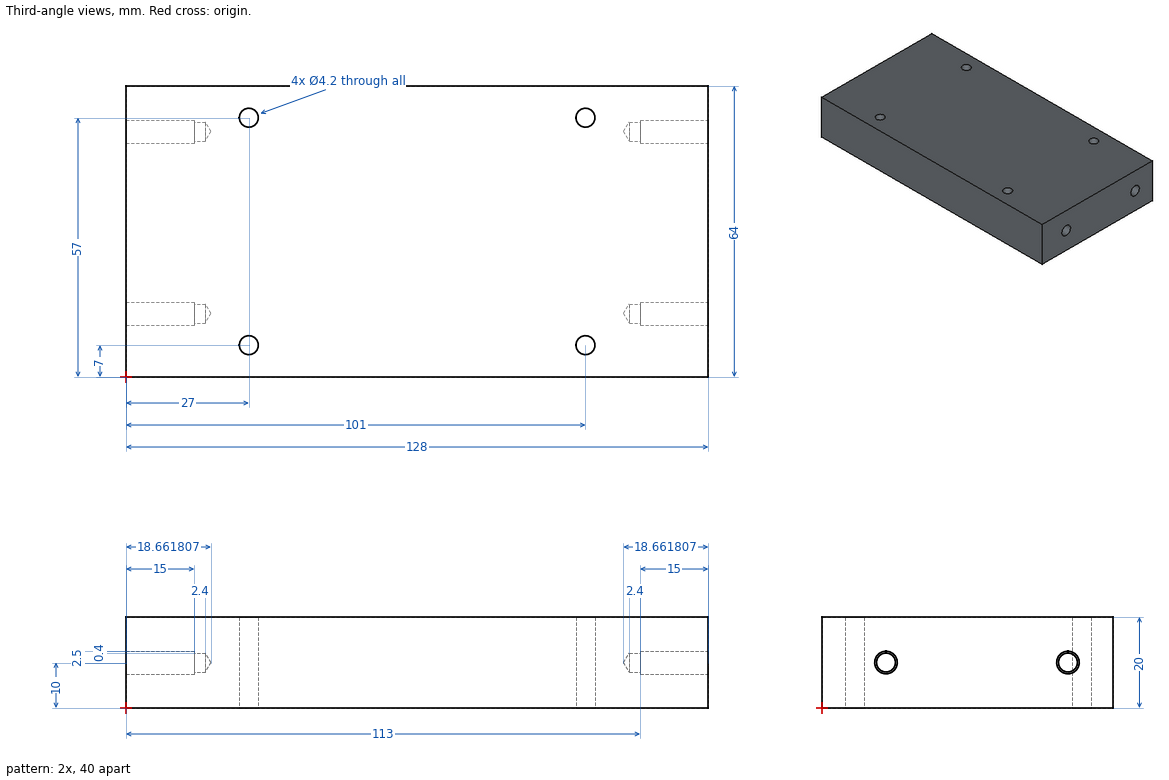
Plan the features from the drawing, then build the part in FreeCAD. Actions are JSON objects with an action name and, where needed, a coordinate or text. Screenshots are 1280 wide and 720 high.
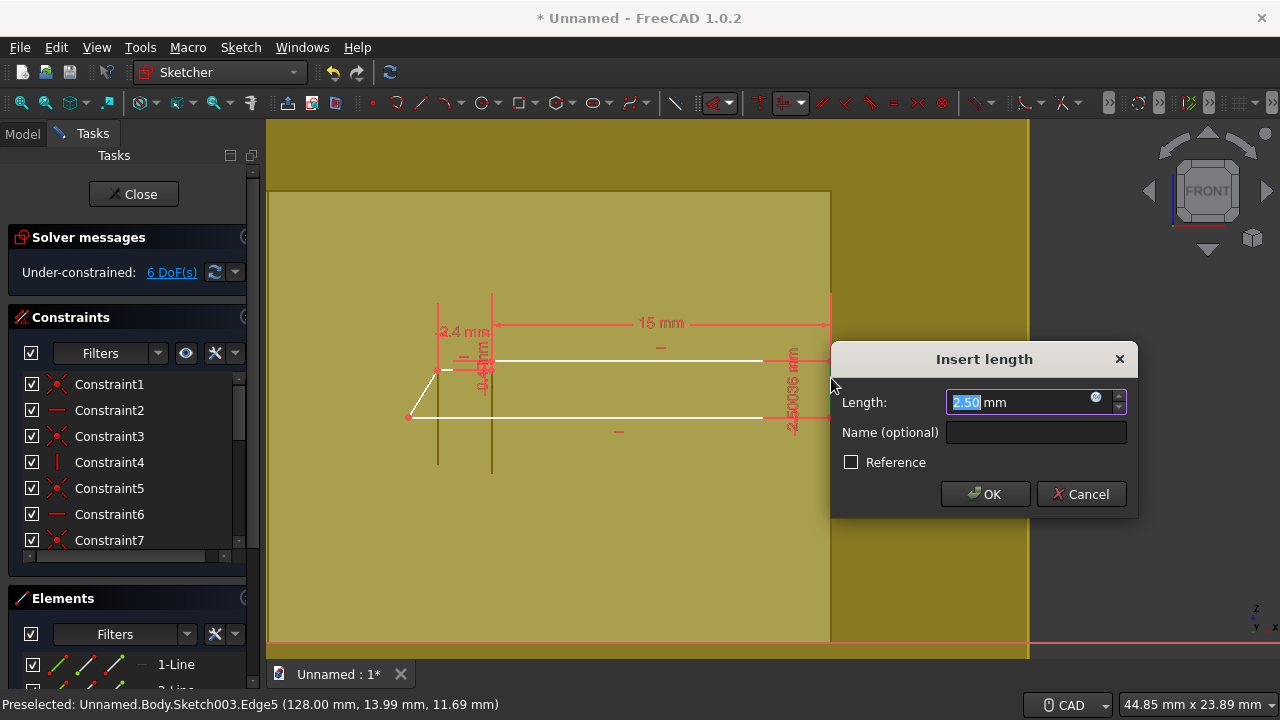
{"action": "type", "text": "2.5"}
{"action": "key", "text": "Return"}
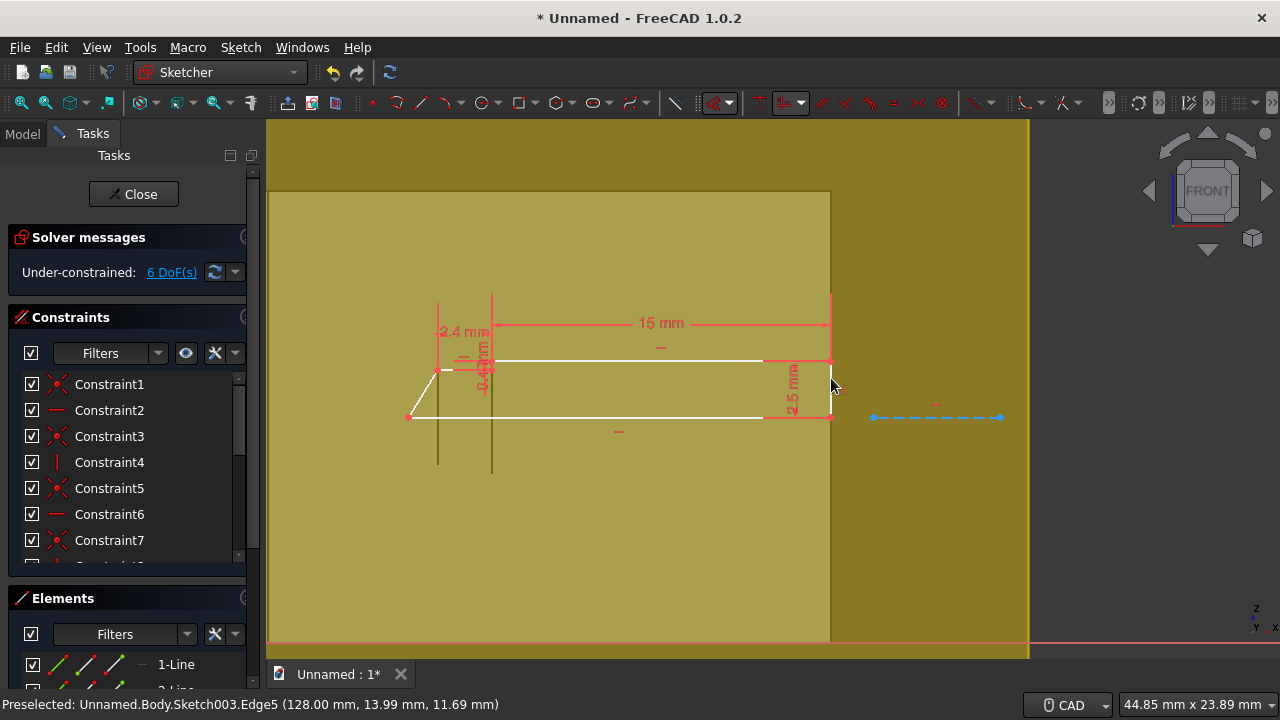
{"action": "left_click", "coordinate": [409, 418]}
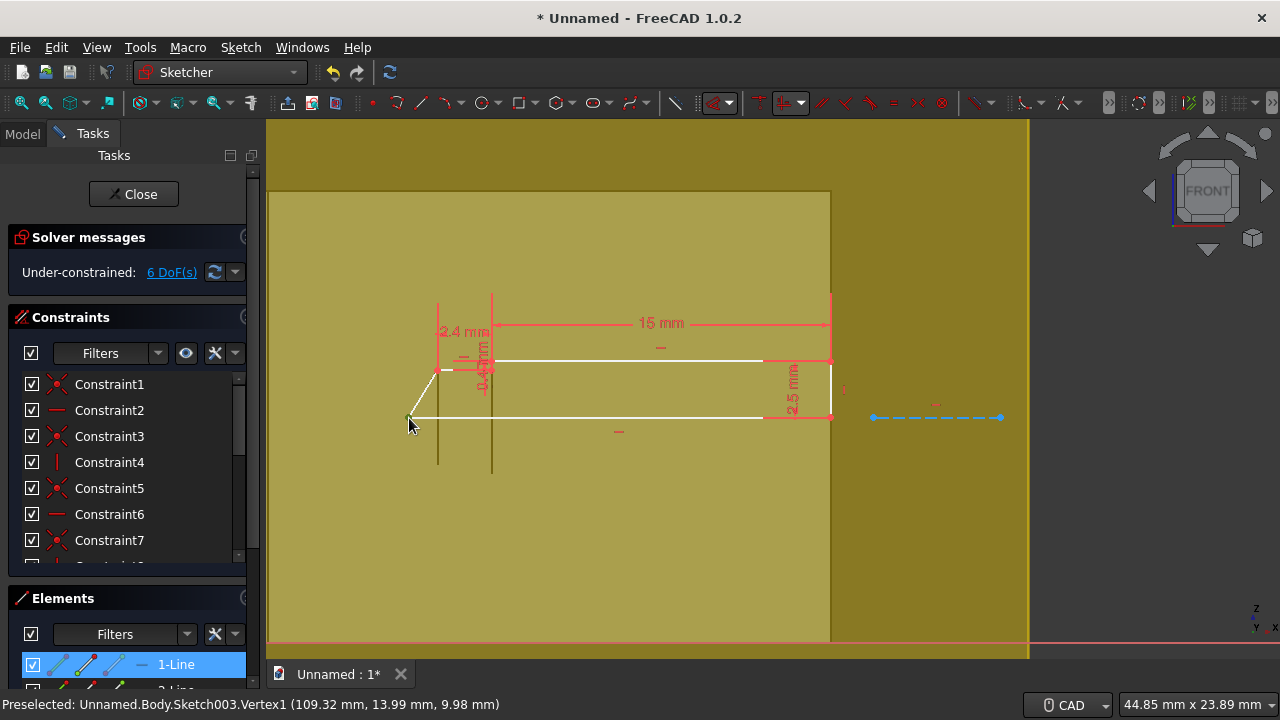
{"action": "left_click", "coordinate": [732, 104]}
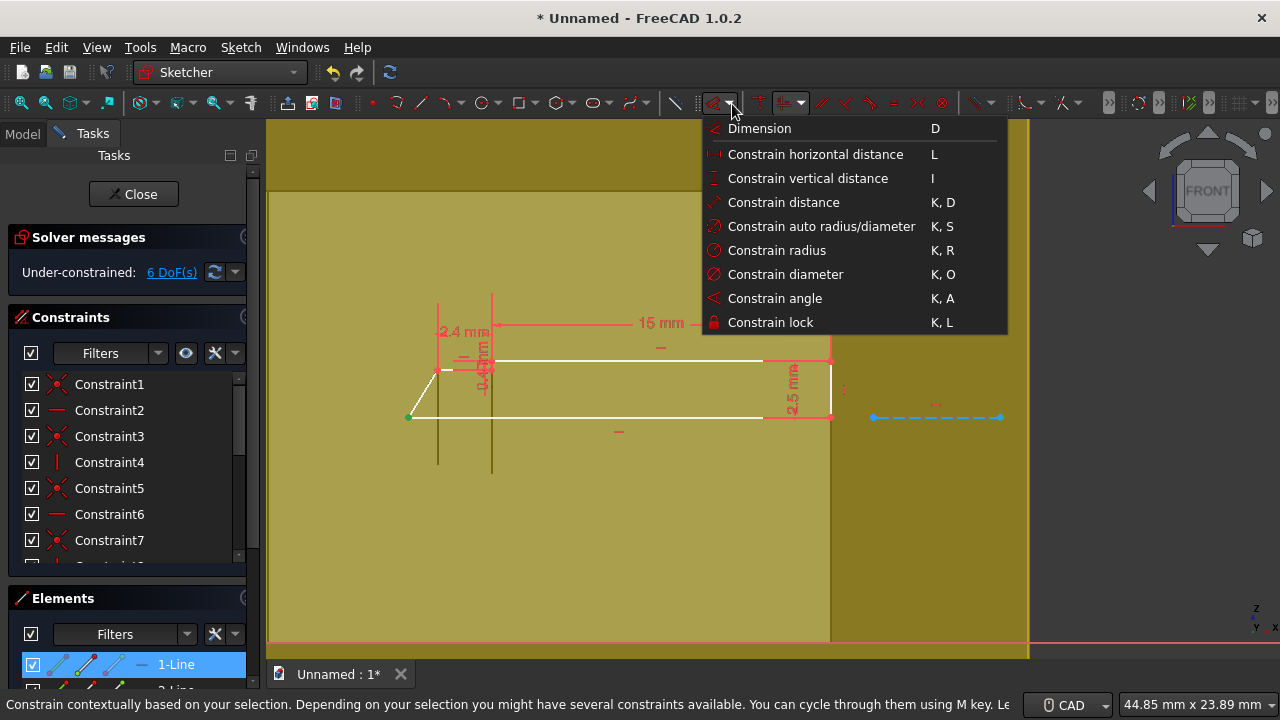
{"action": "left_click", "coordinate": [855, 178]}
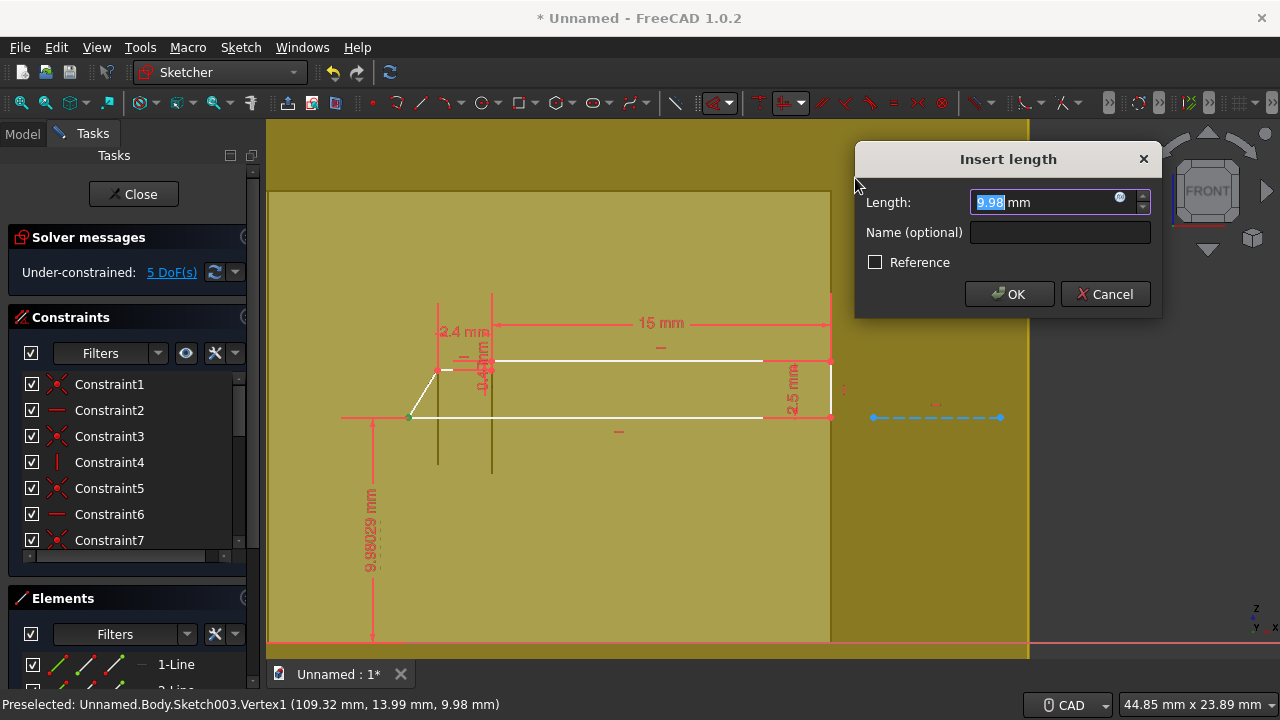
{"action": "type", "text": "10"}
{"action": "key", "text": "Return"}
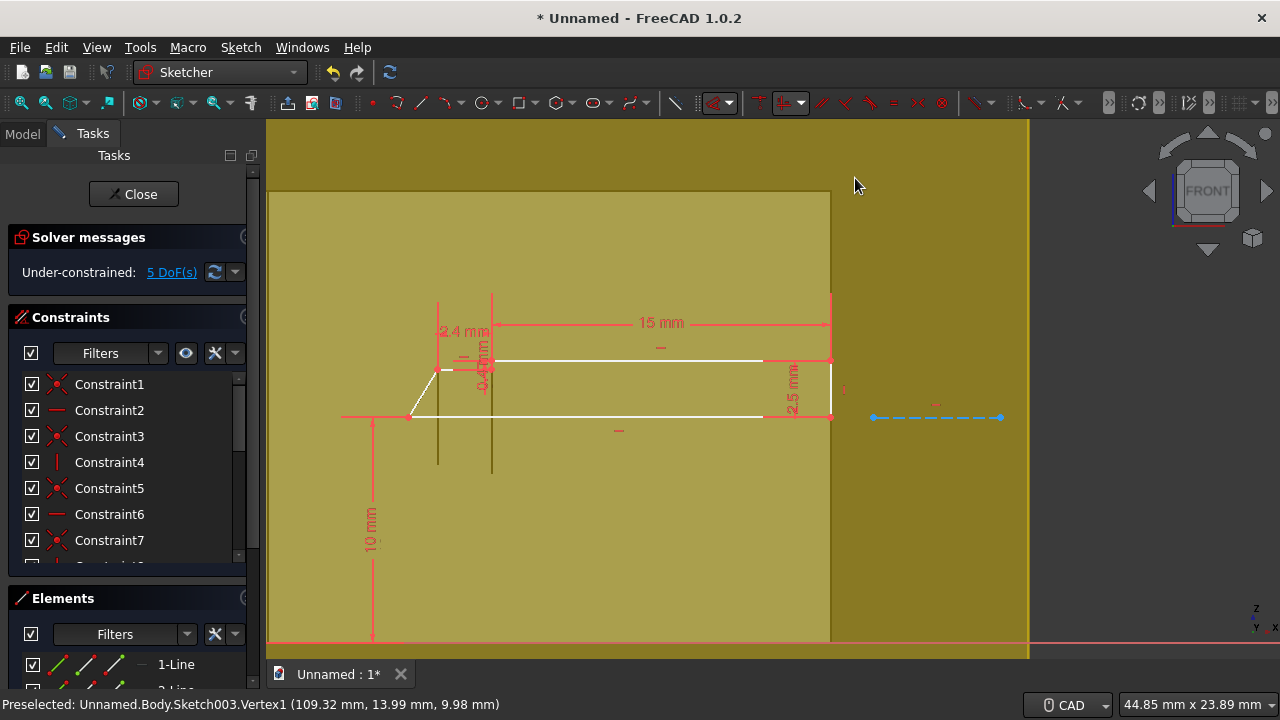
{"action": "left_click", "coordinate": [873, 418]}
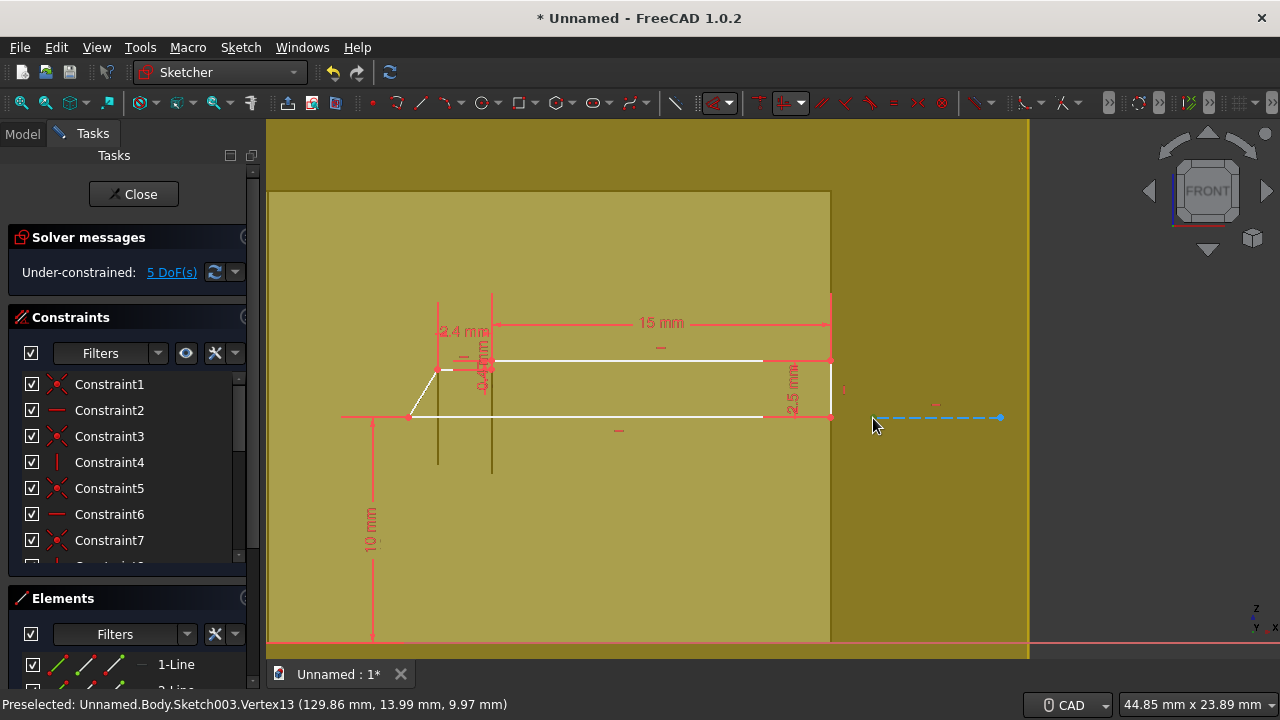
{"action": "left_click", "coordinate": [732, 104]}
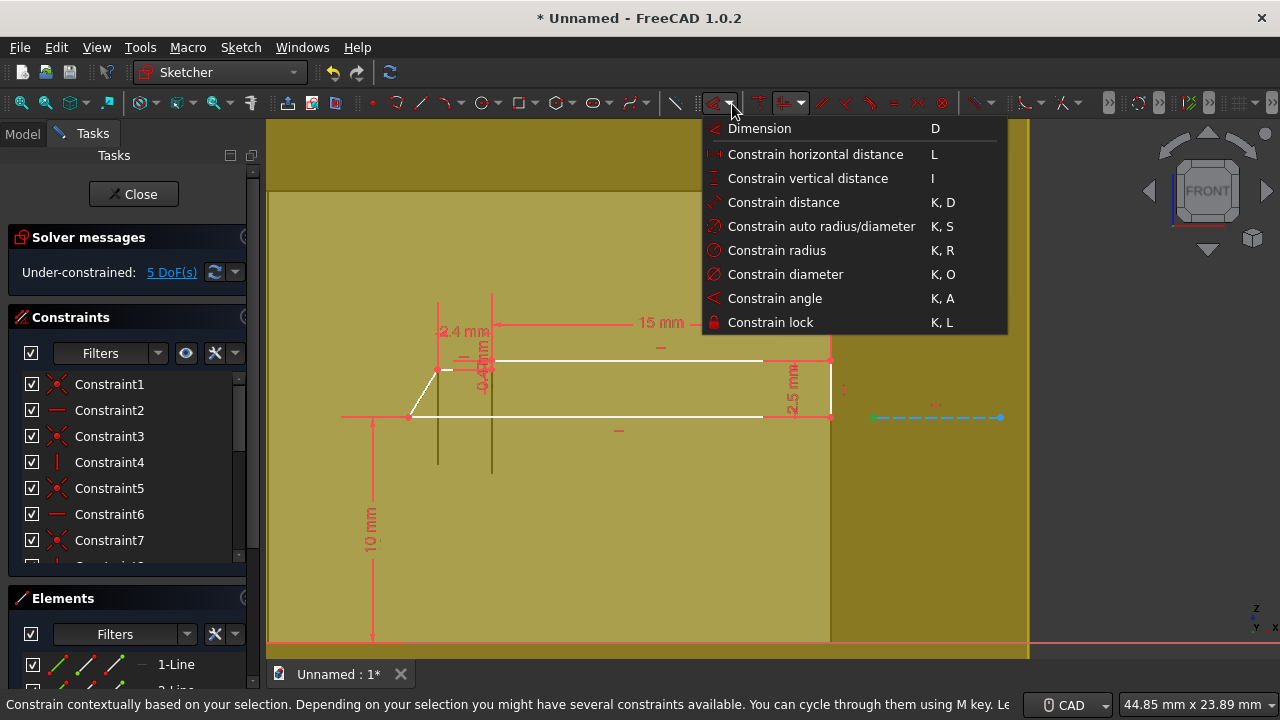
{"action": "left_click", "coordinate": [855, 178]}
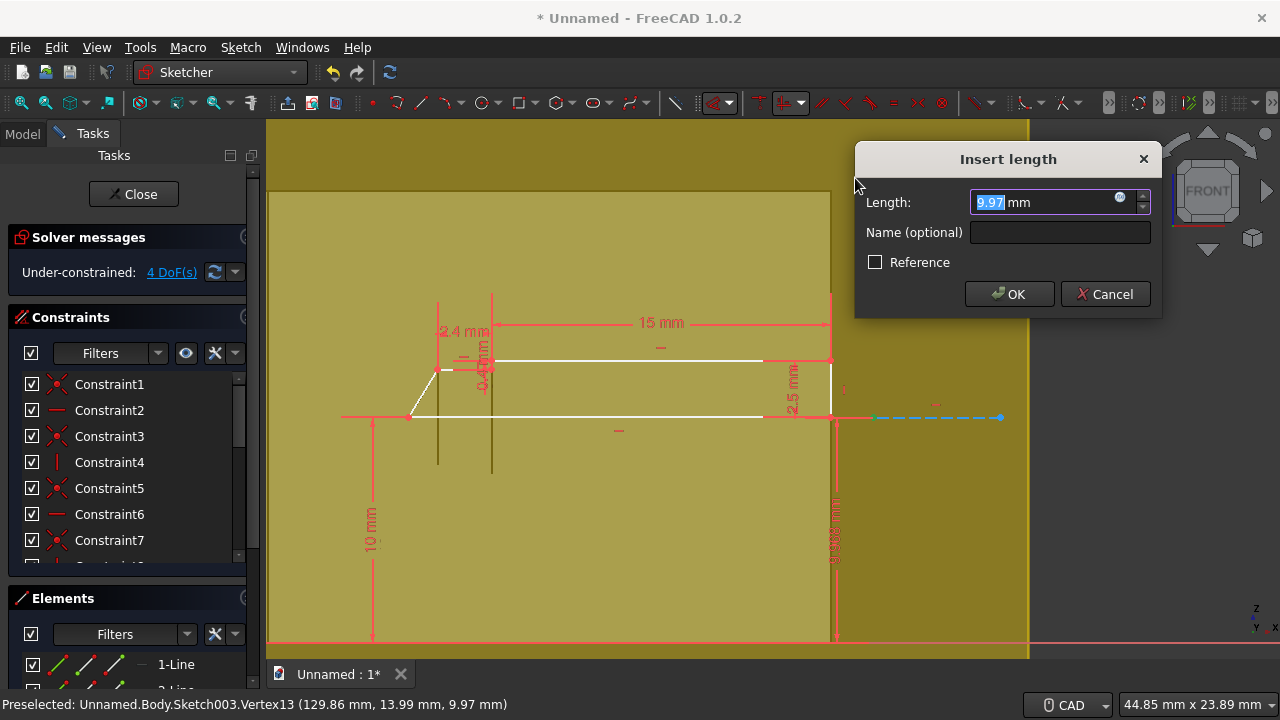
{"action": "type", "text": "10"}
{"action": "key", "text": "Return"}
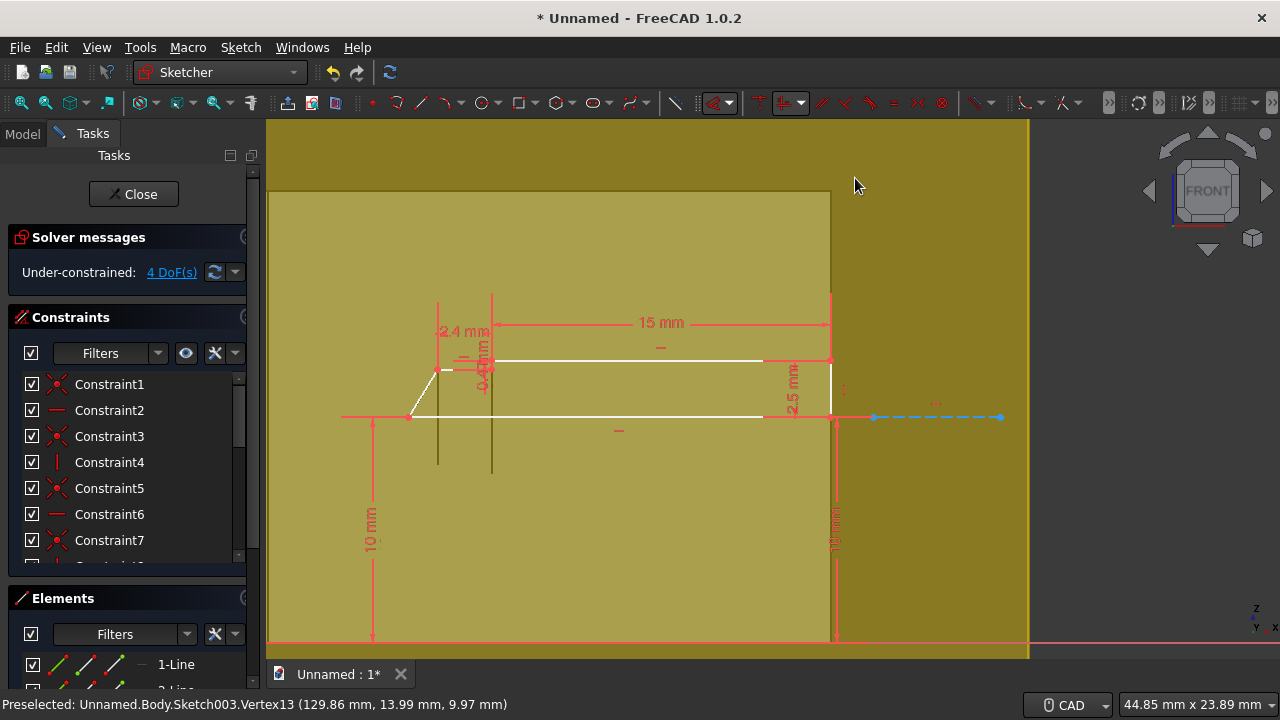
{"action": "scroll", "coordinate": [492, 370], "scroll_direction": "up", "scroll_amount": 2}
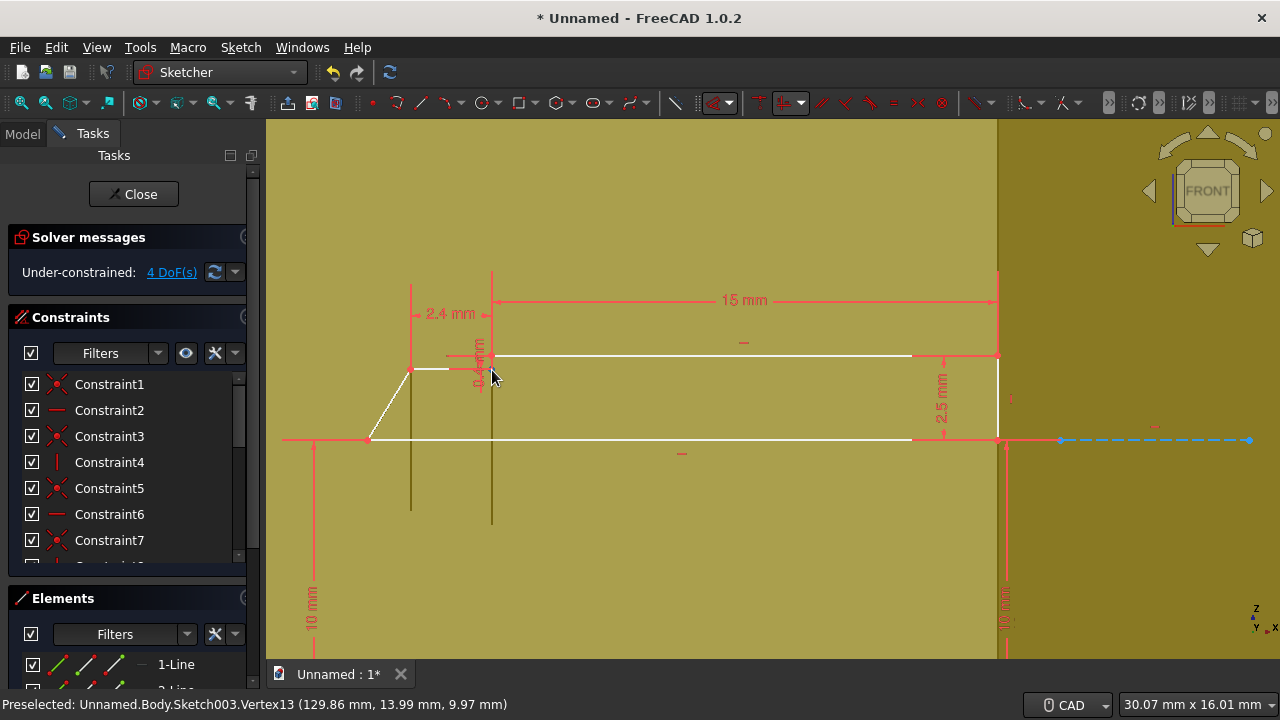
{"action": "left_click", "coordinate": [492, 369]}